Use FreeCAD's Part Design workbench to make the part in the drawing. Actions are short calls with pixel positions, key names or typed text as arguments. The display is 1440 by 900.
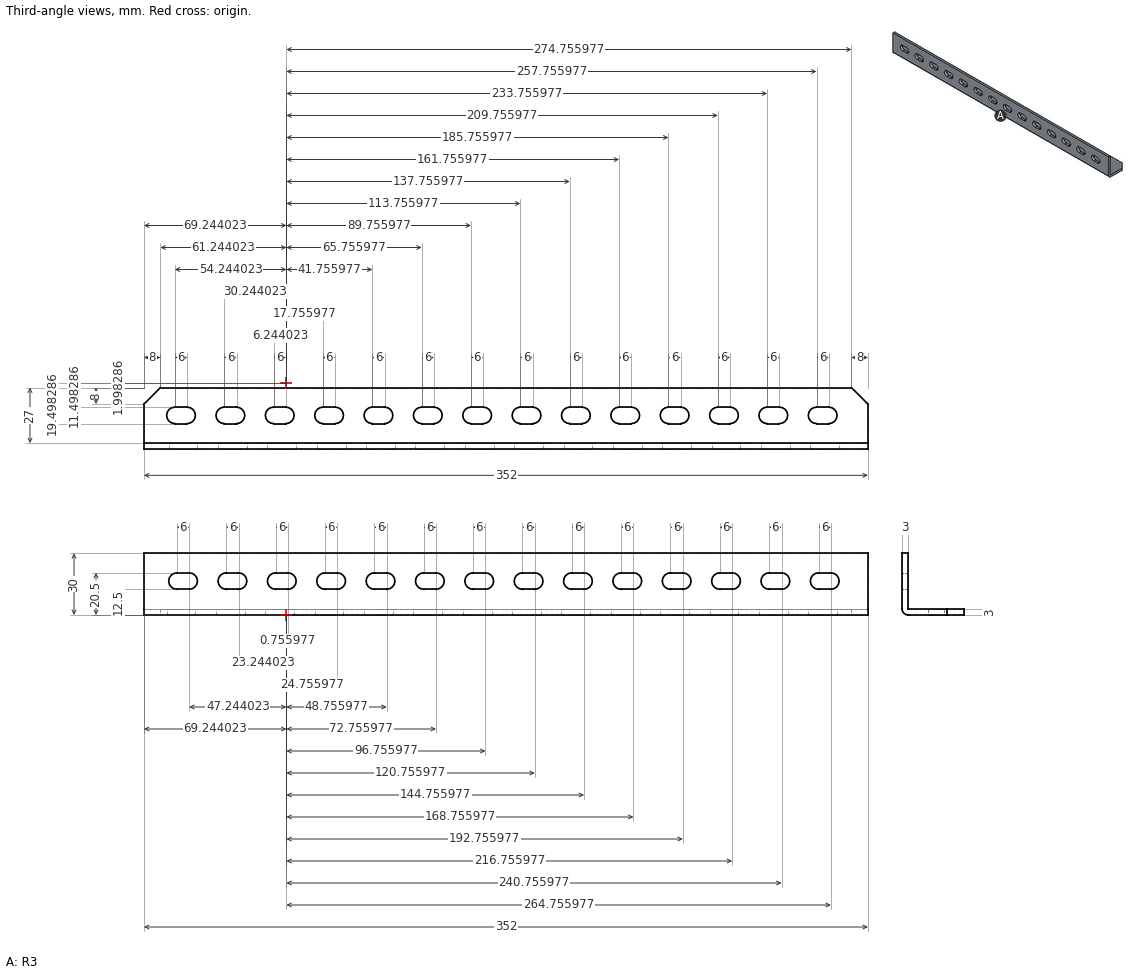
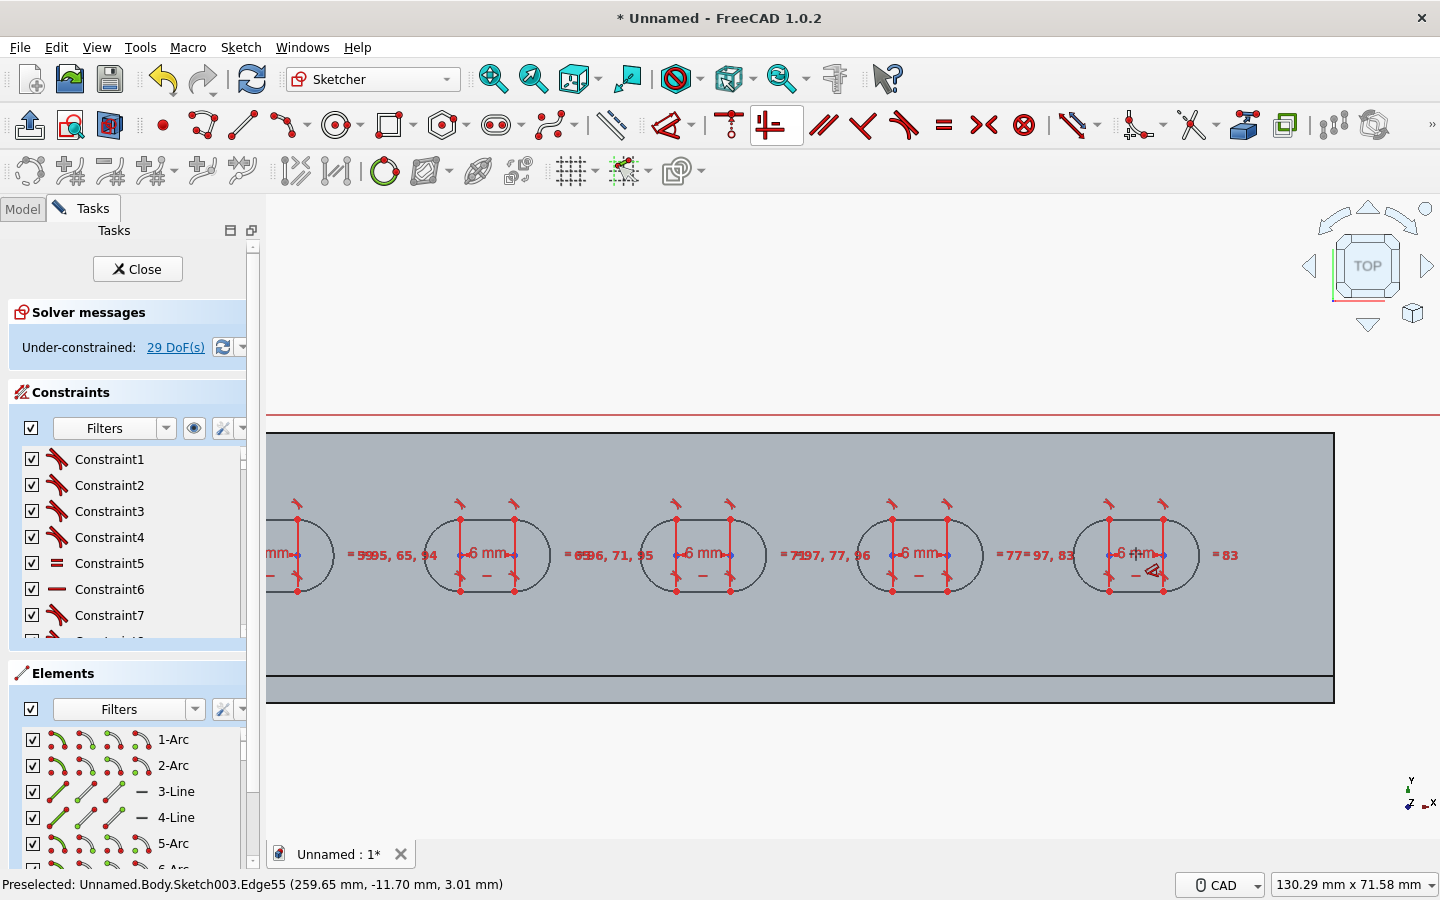
scroll(1130, 521, down, 7)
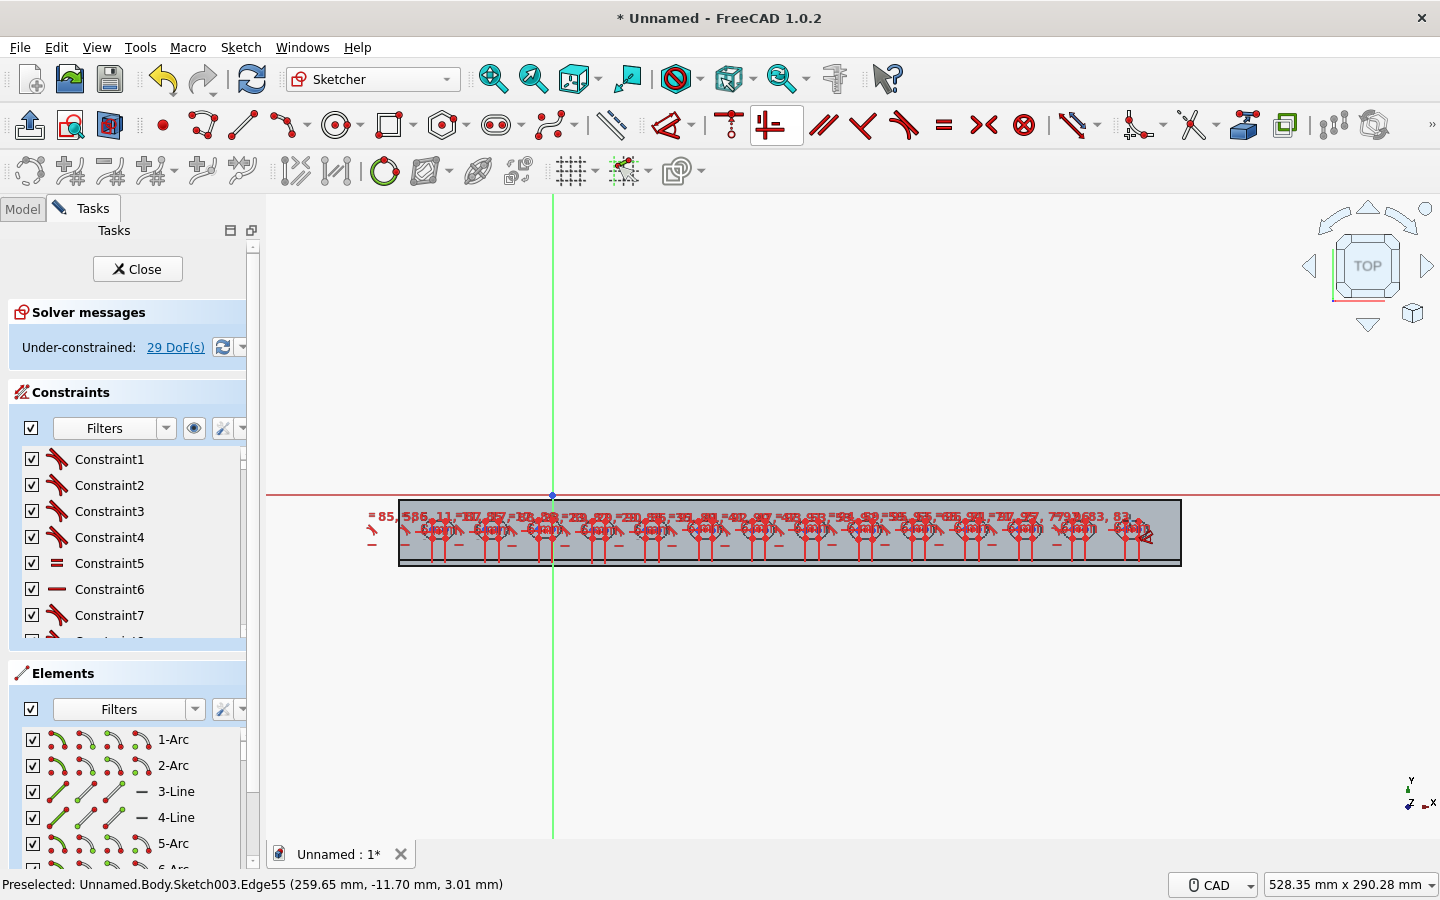
scroll(539, 521, up, 6)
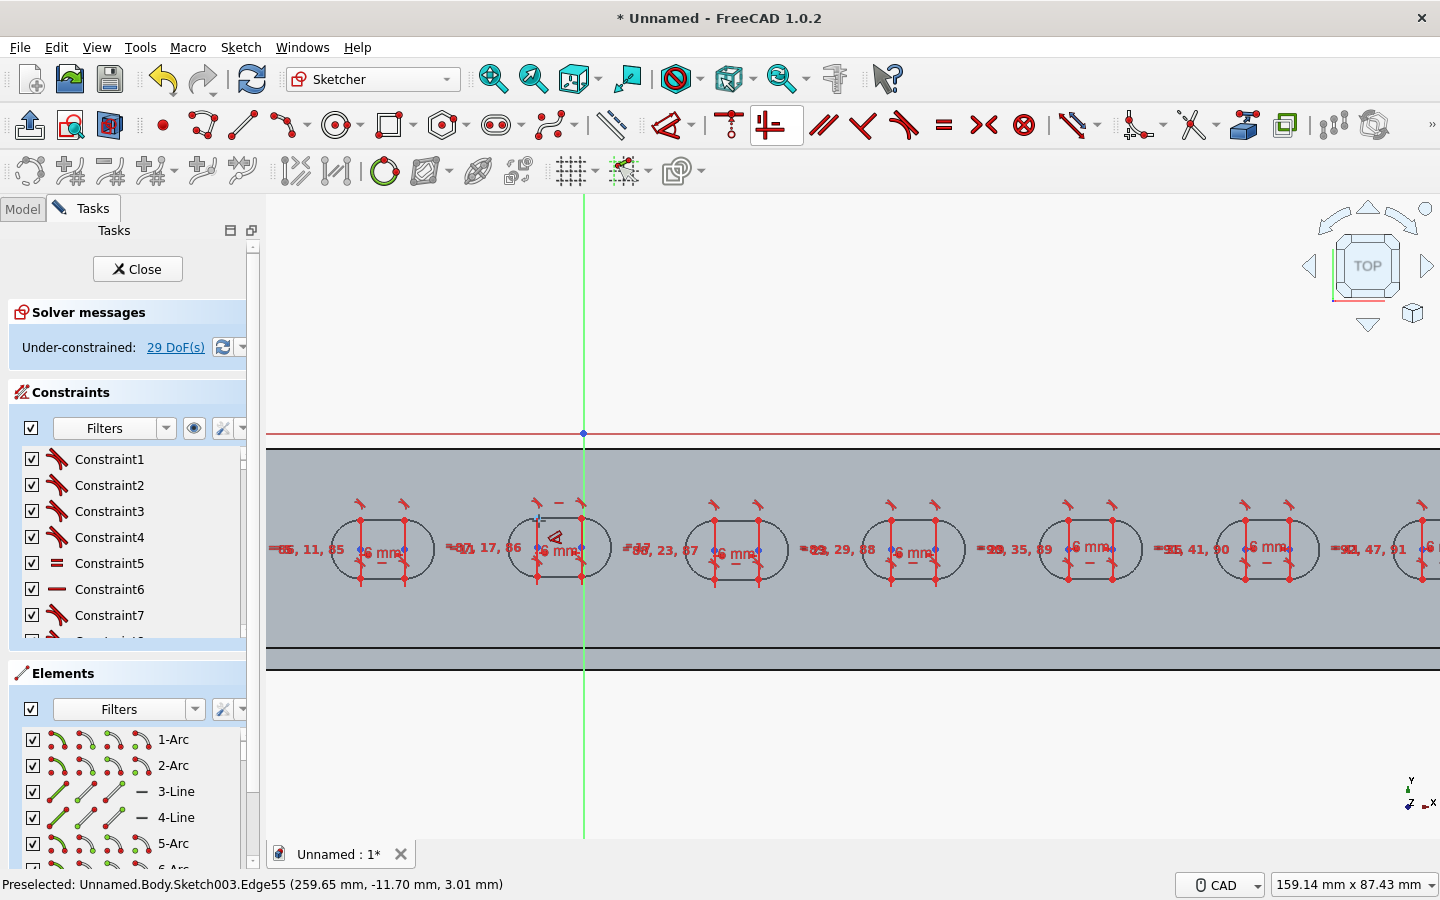
click(537, 518)
click(561, 400)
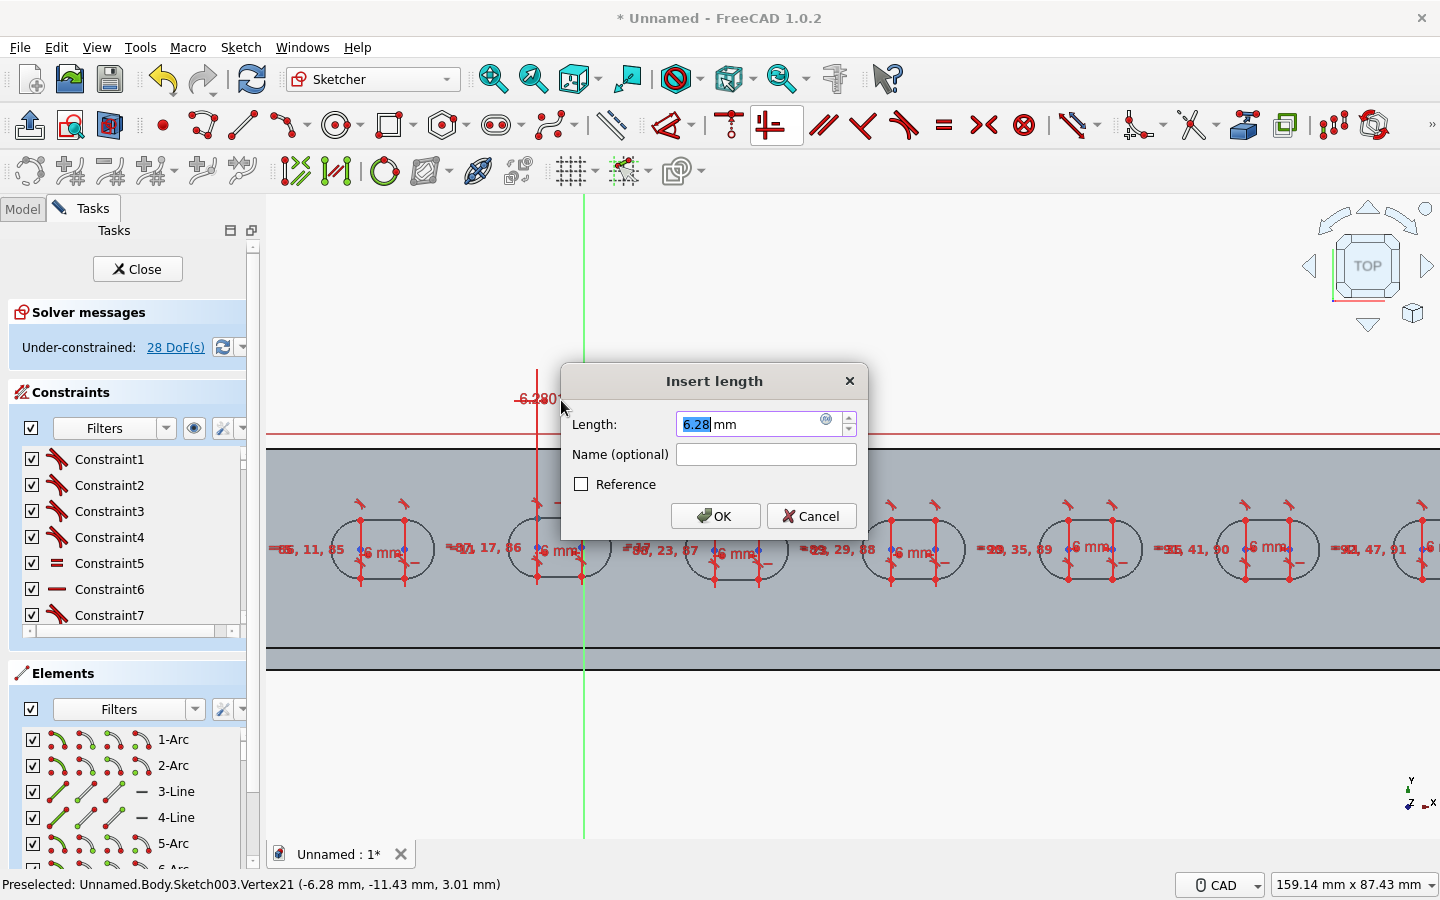
text(6.244023)
key(Return)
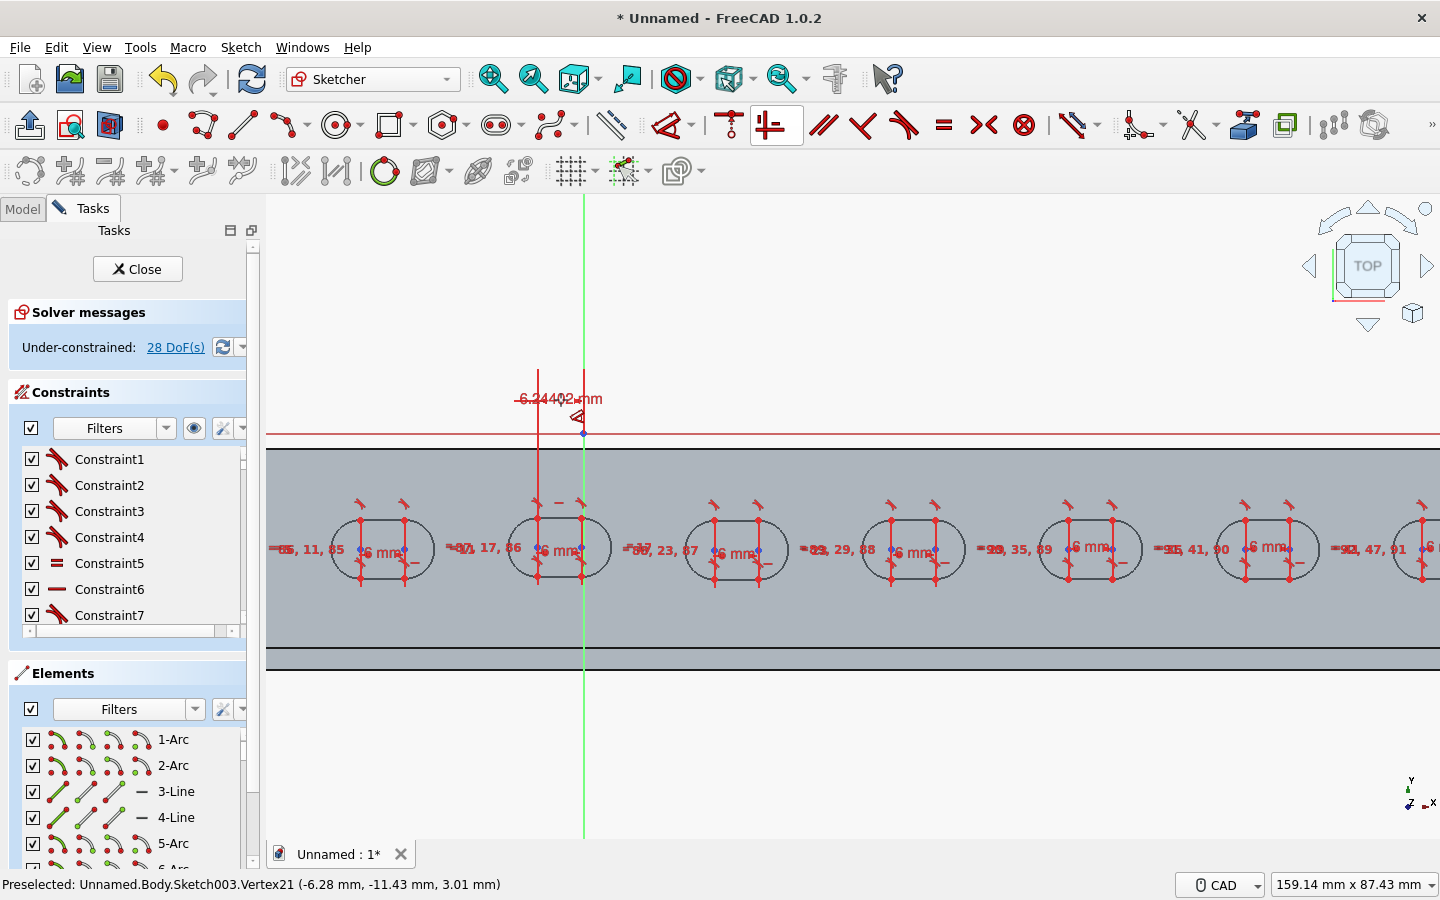
scroll(538, 521, down, 6)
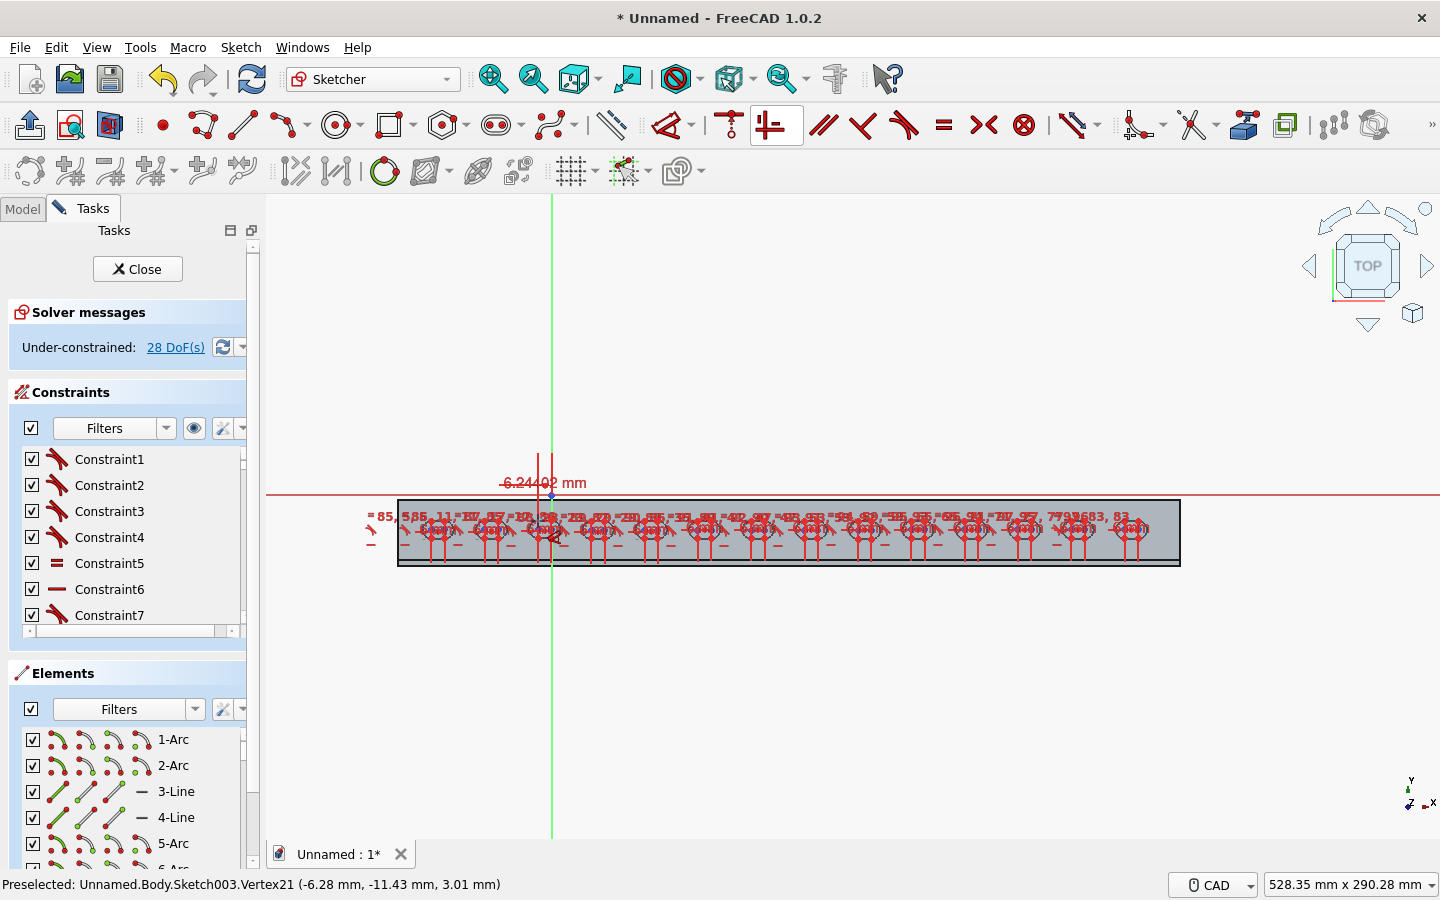
scroll(431, 521, up, 2)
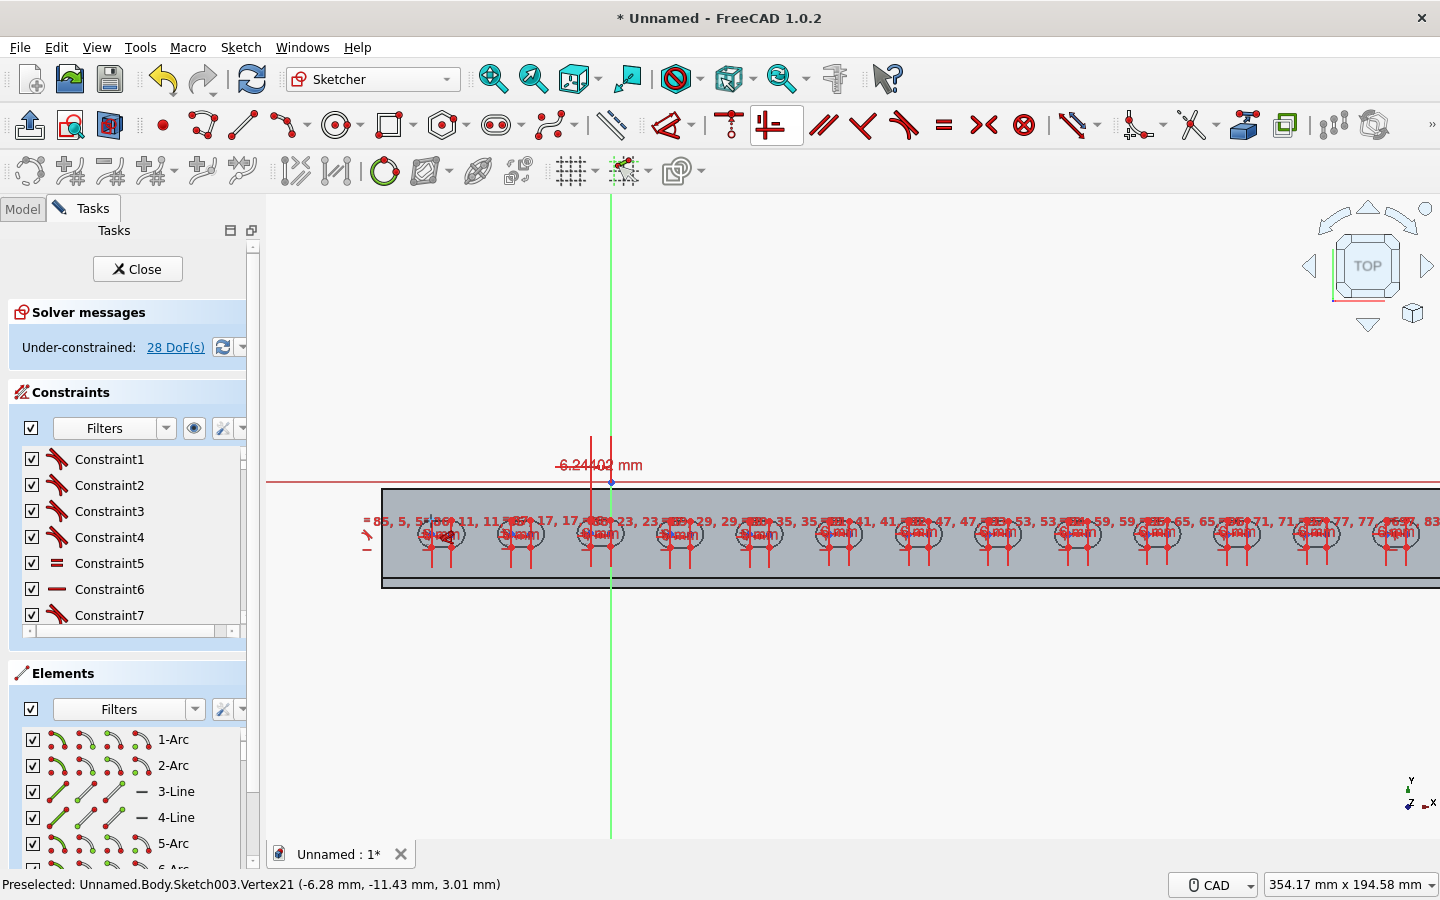
click(432, 521)
click(521, 448)